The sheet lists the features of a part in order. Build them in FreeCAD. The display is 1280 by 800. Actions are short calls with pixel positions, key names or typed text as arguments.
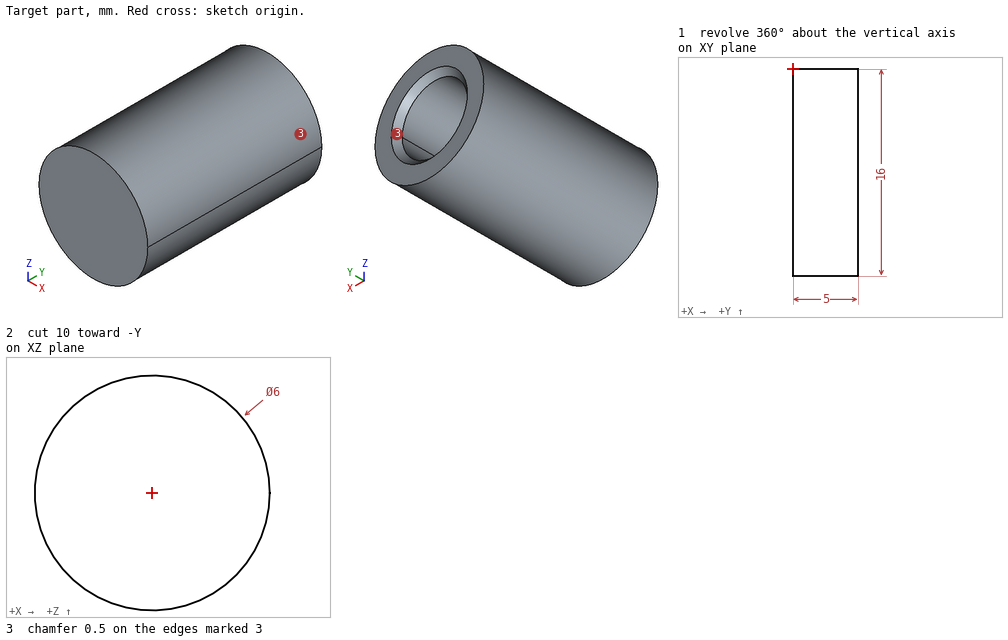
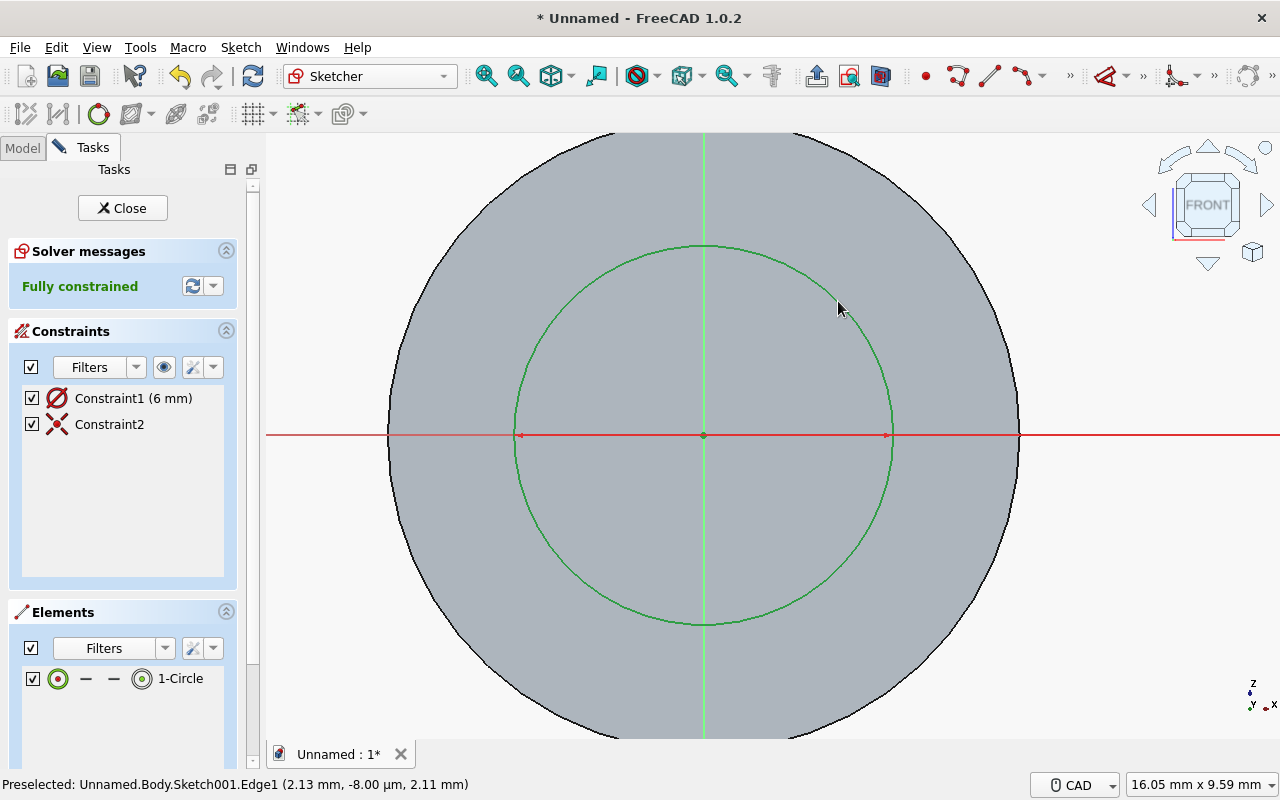
click(123, 208)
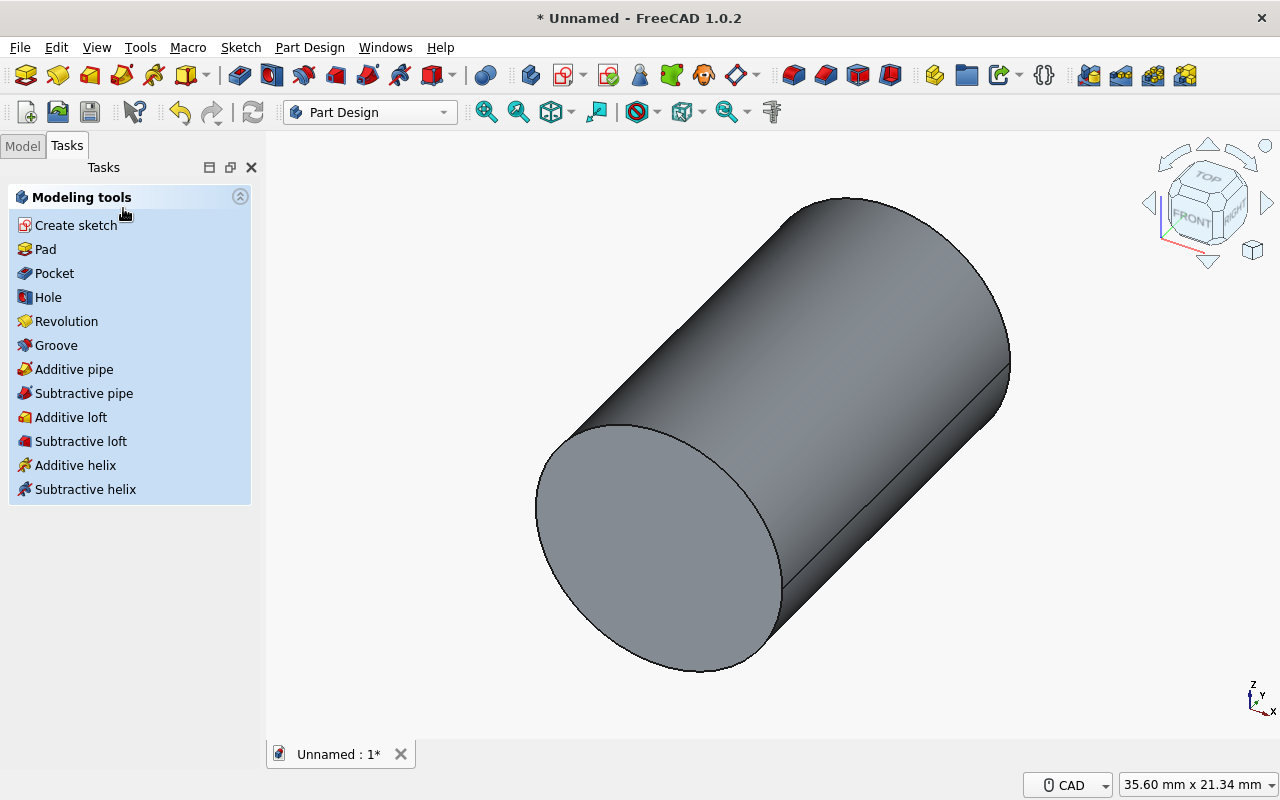
click(240, 76)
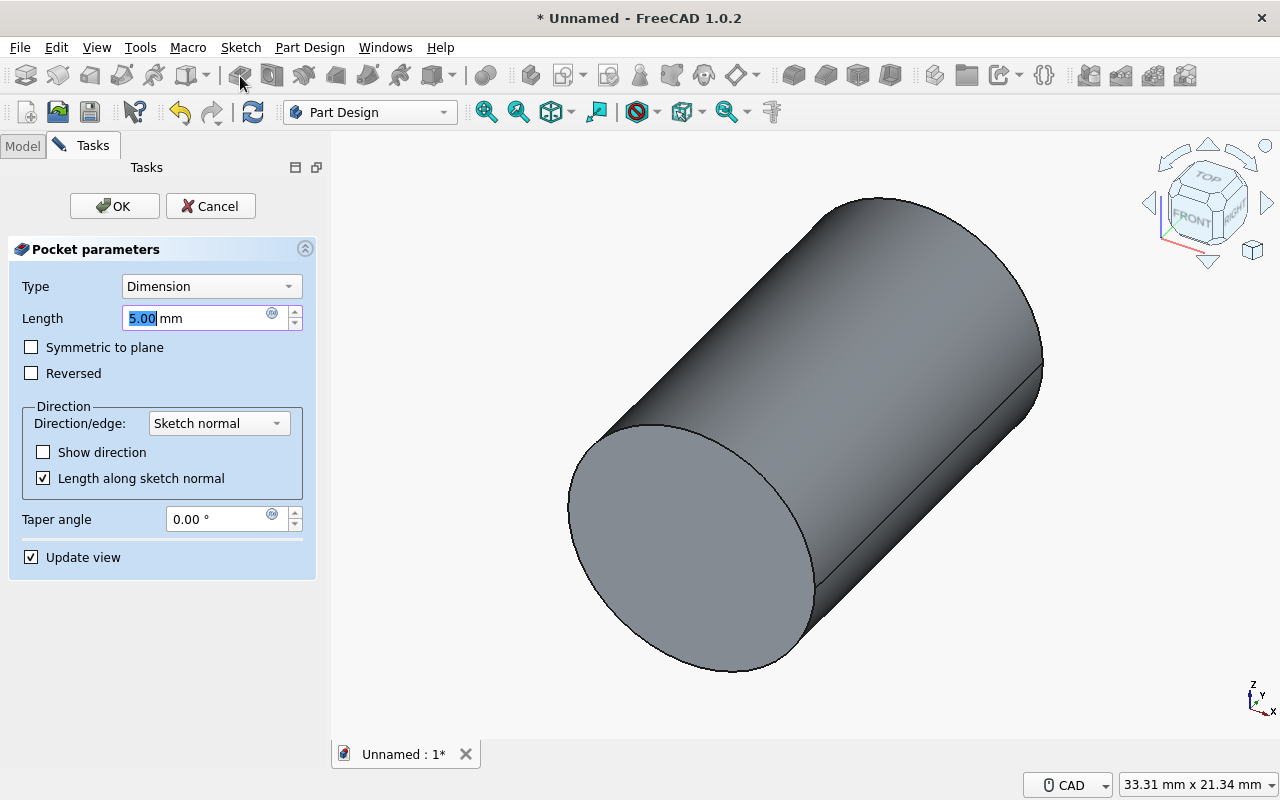
text(10)
key(Tab)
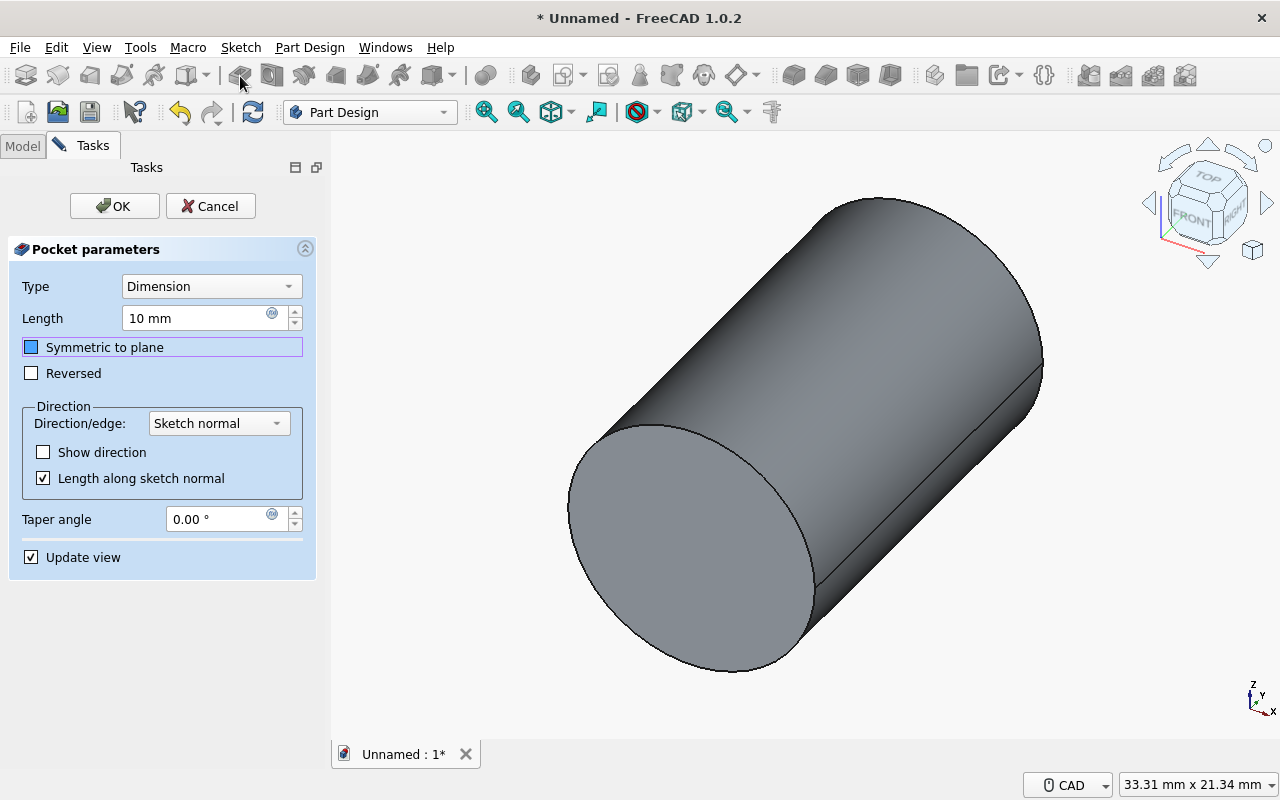
click(30, 373)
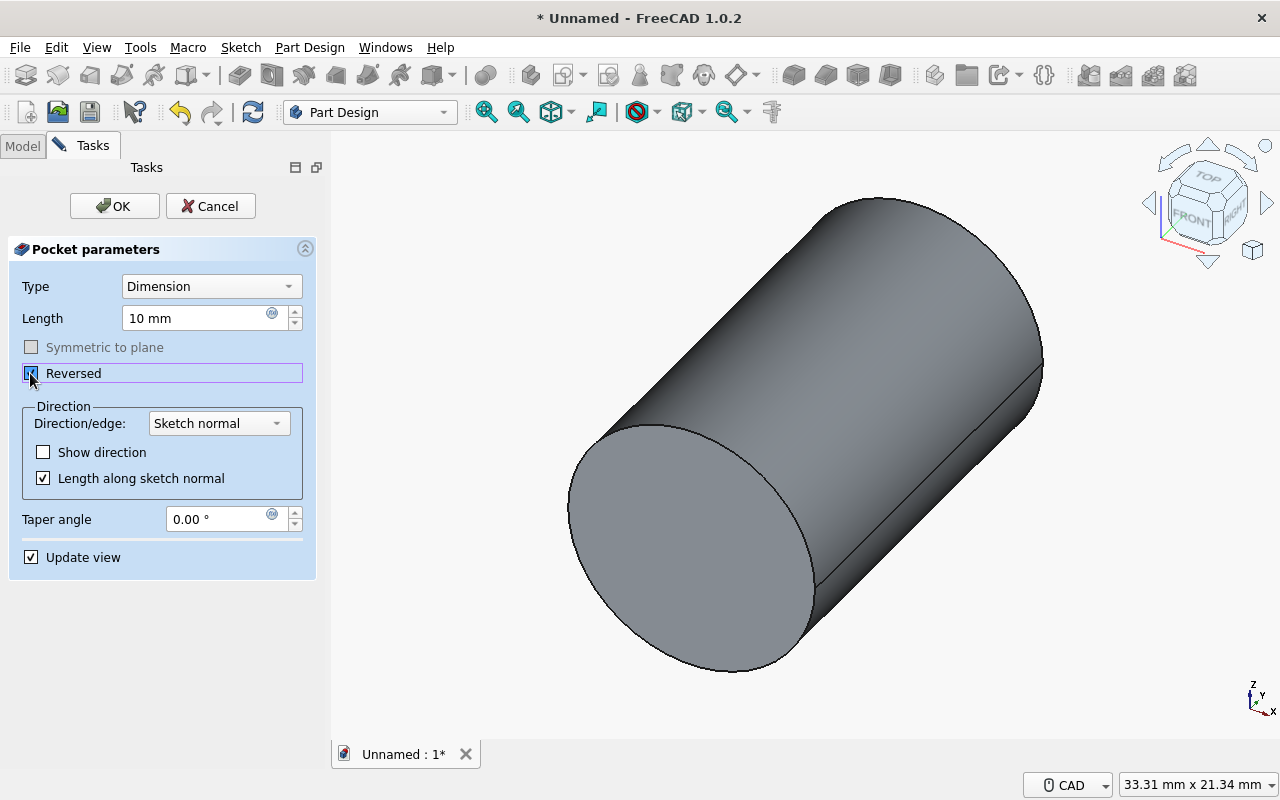
click(115, 206)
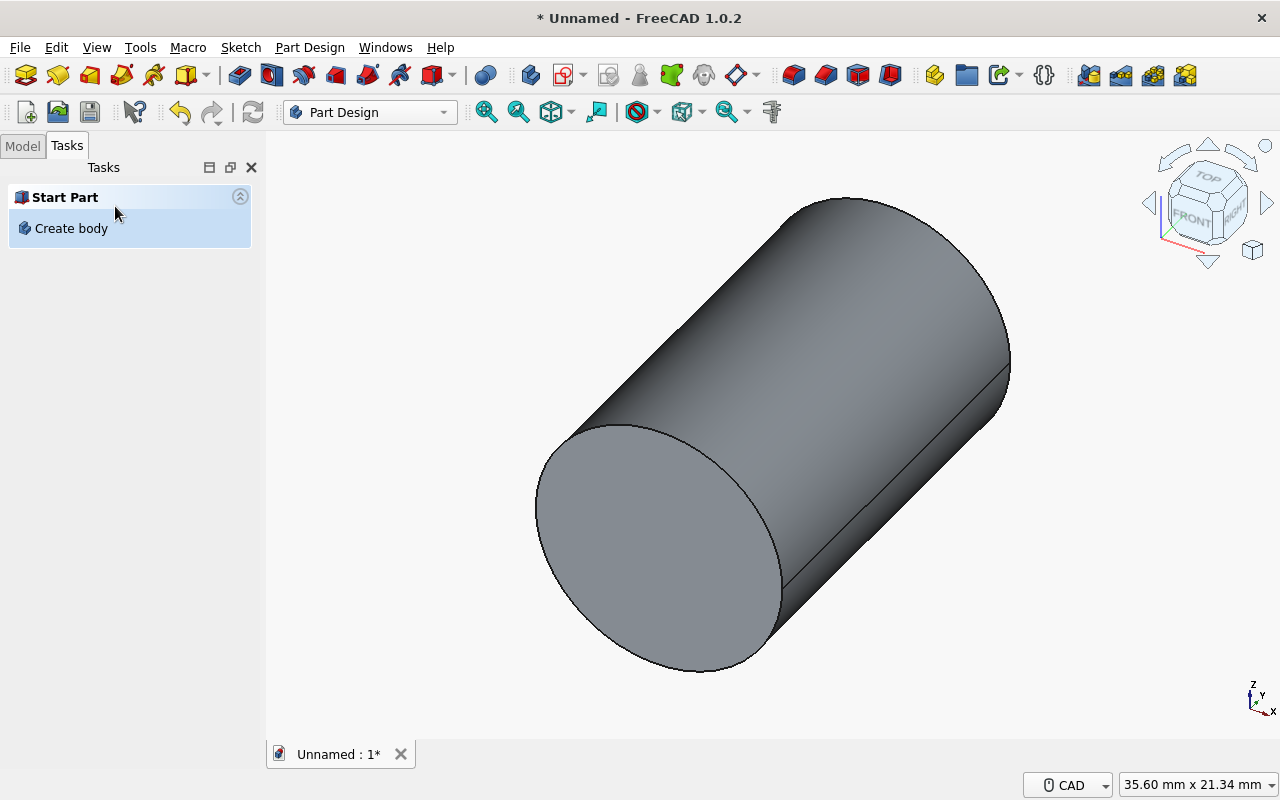
key(0)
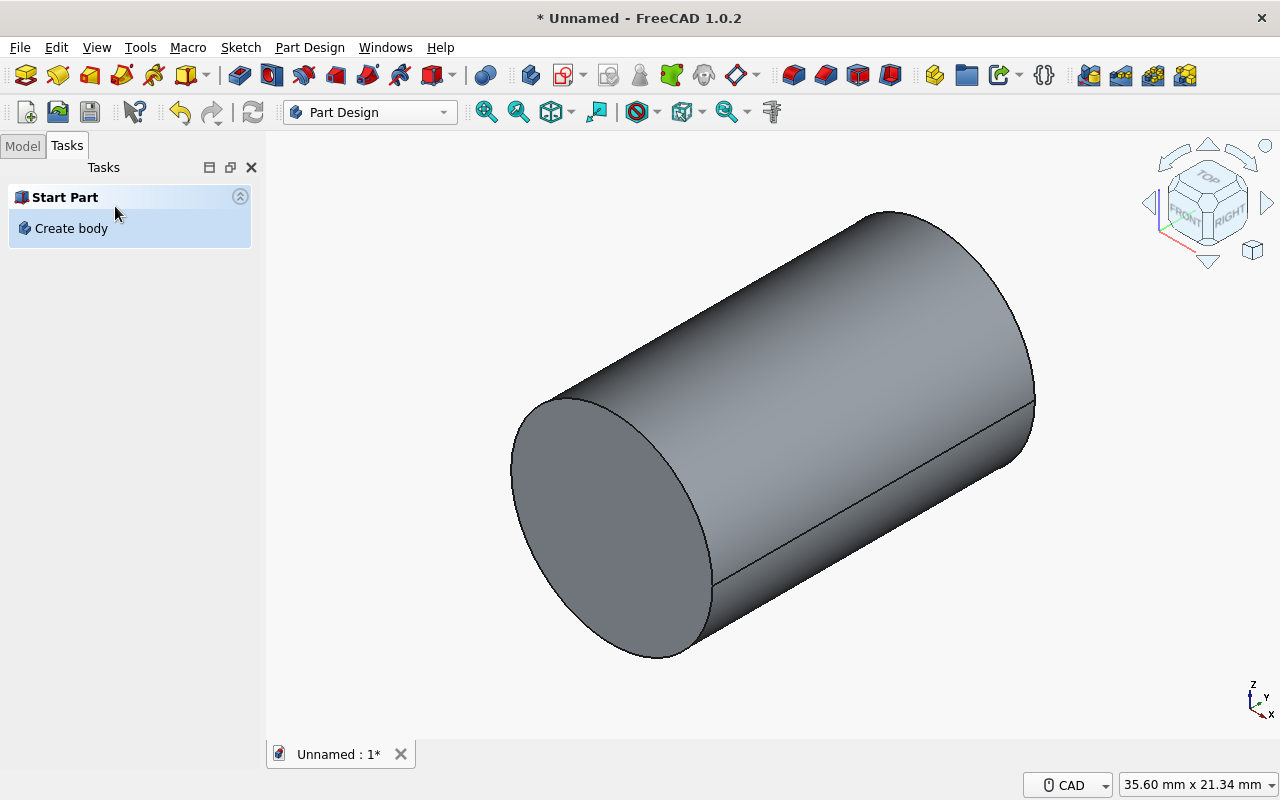
key(2)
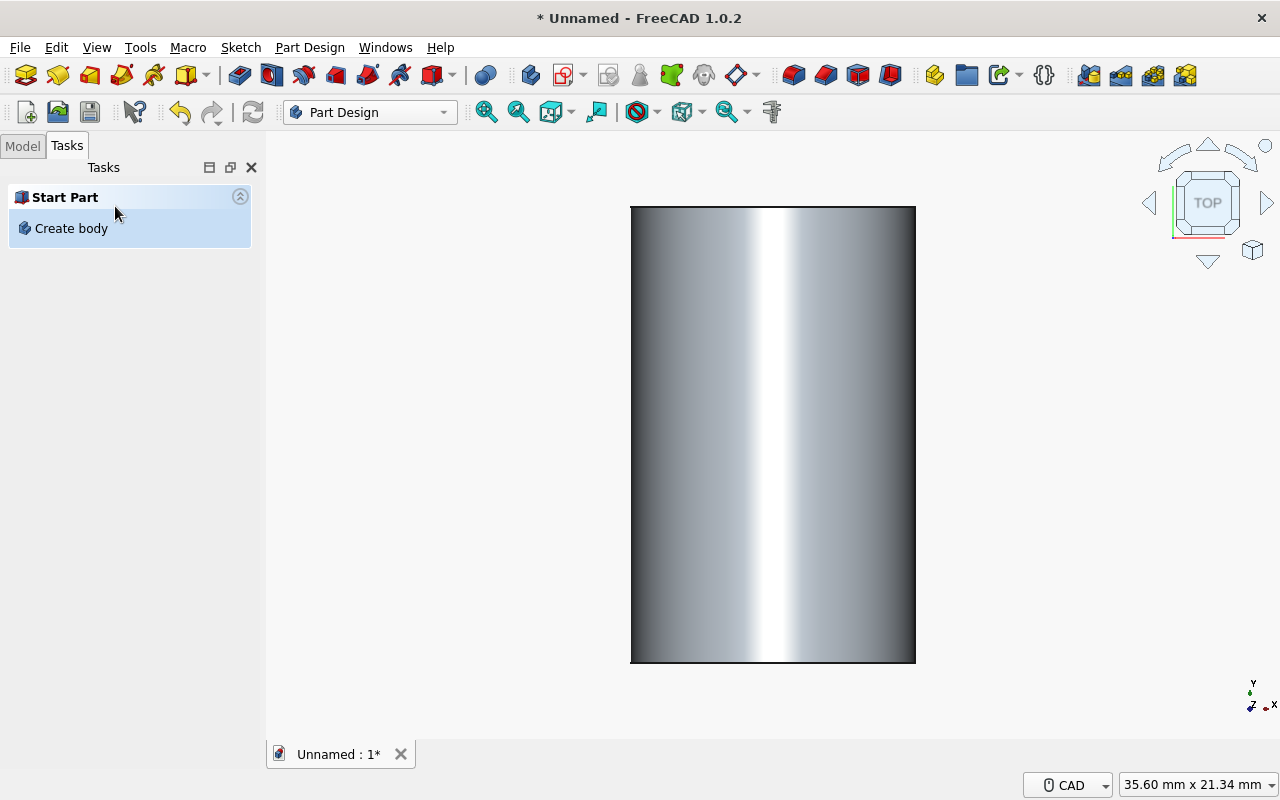
key(1)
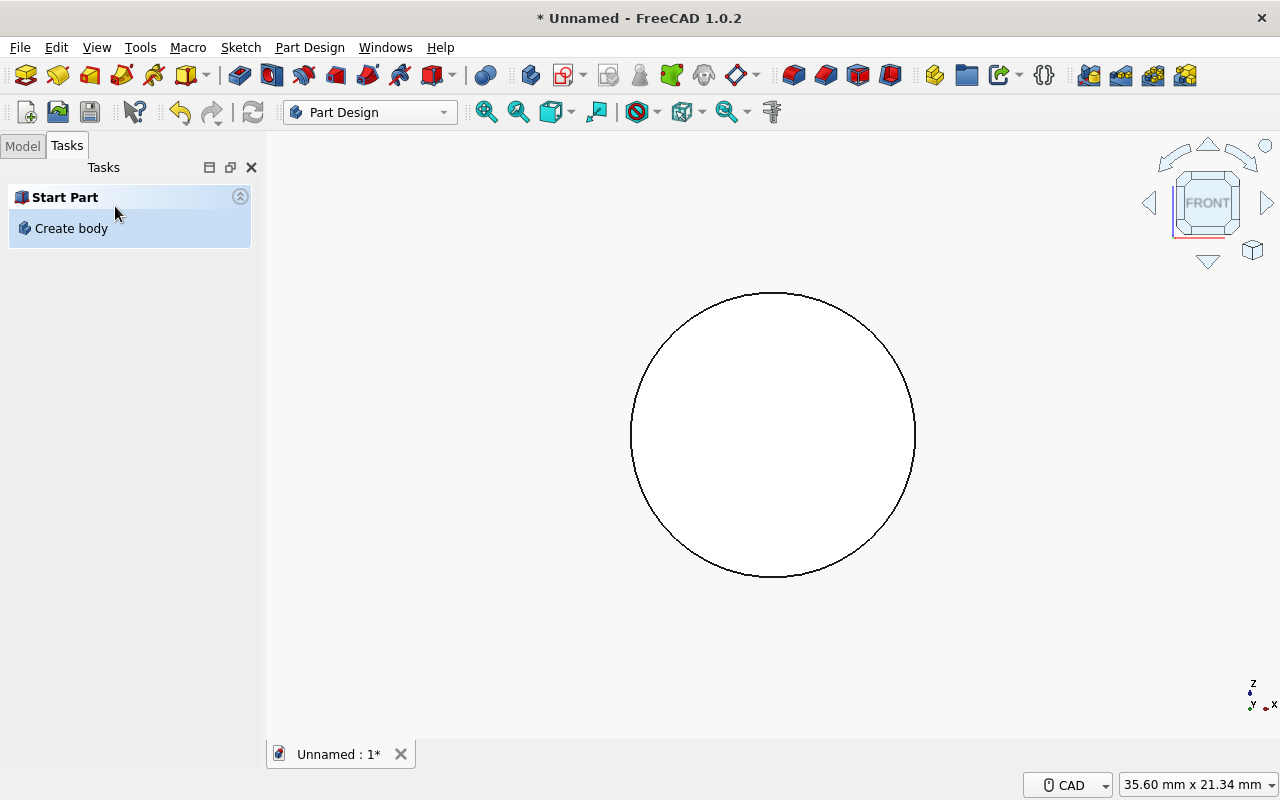
key(3)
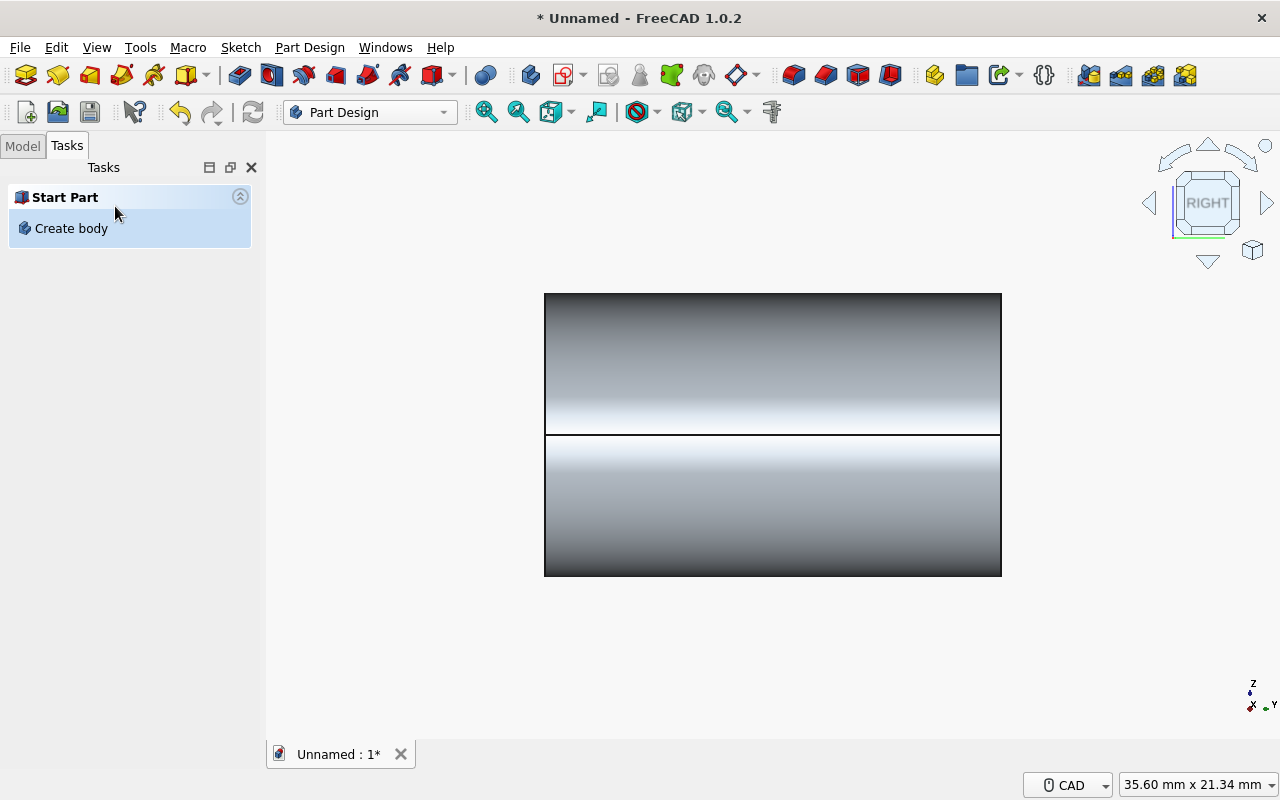
key(5)